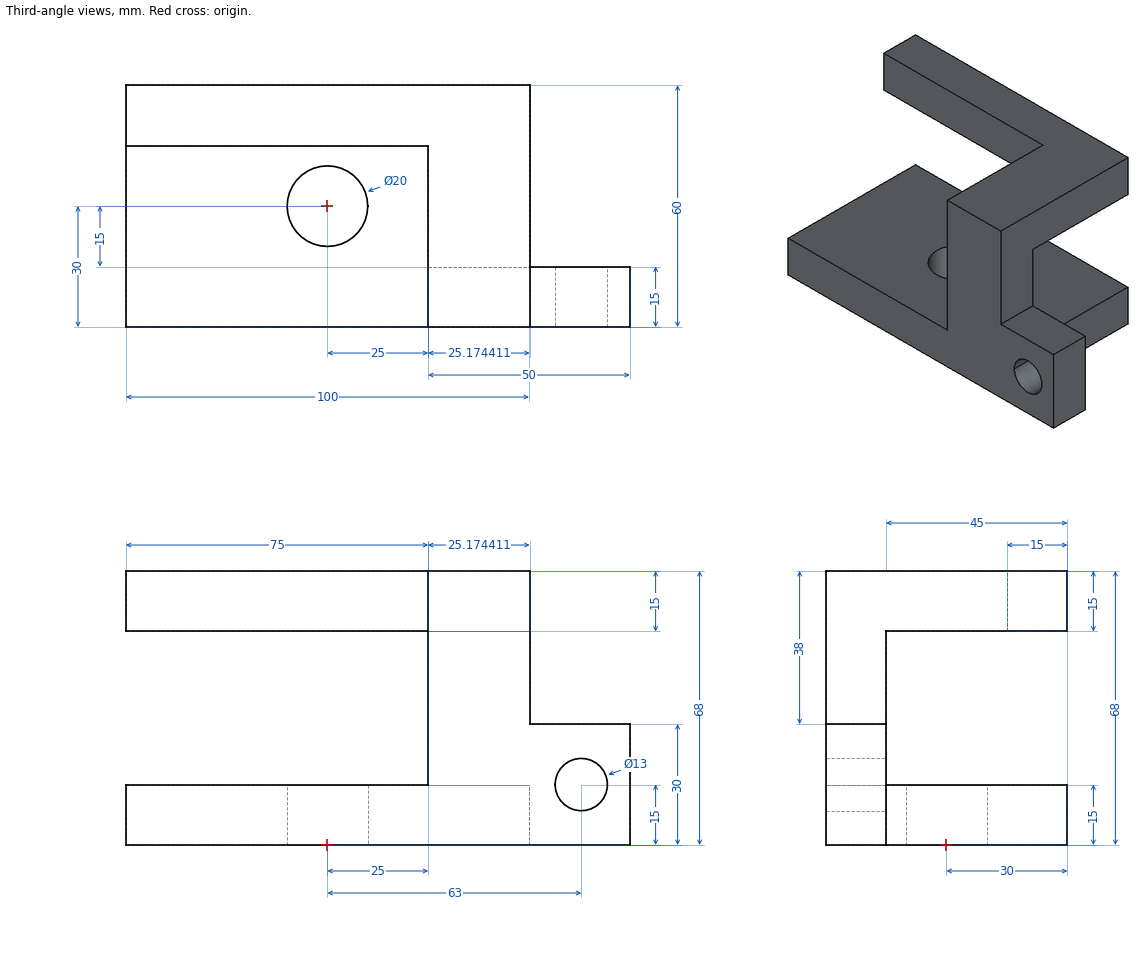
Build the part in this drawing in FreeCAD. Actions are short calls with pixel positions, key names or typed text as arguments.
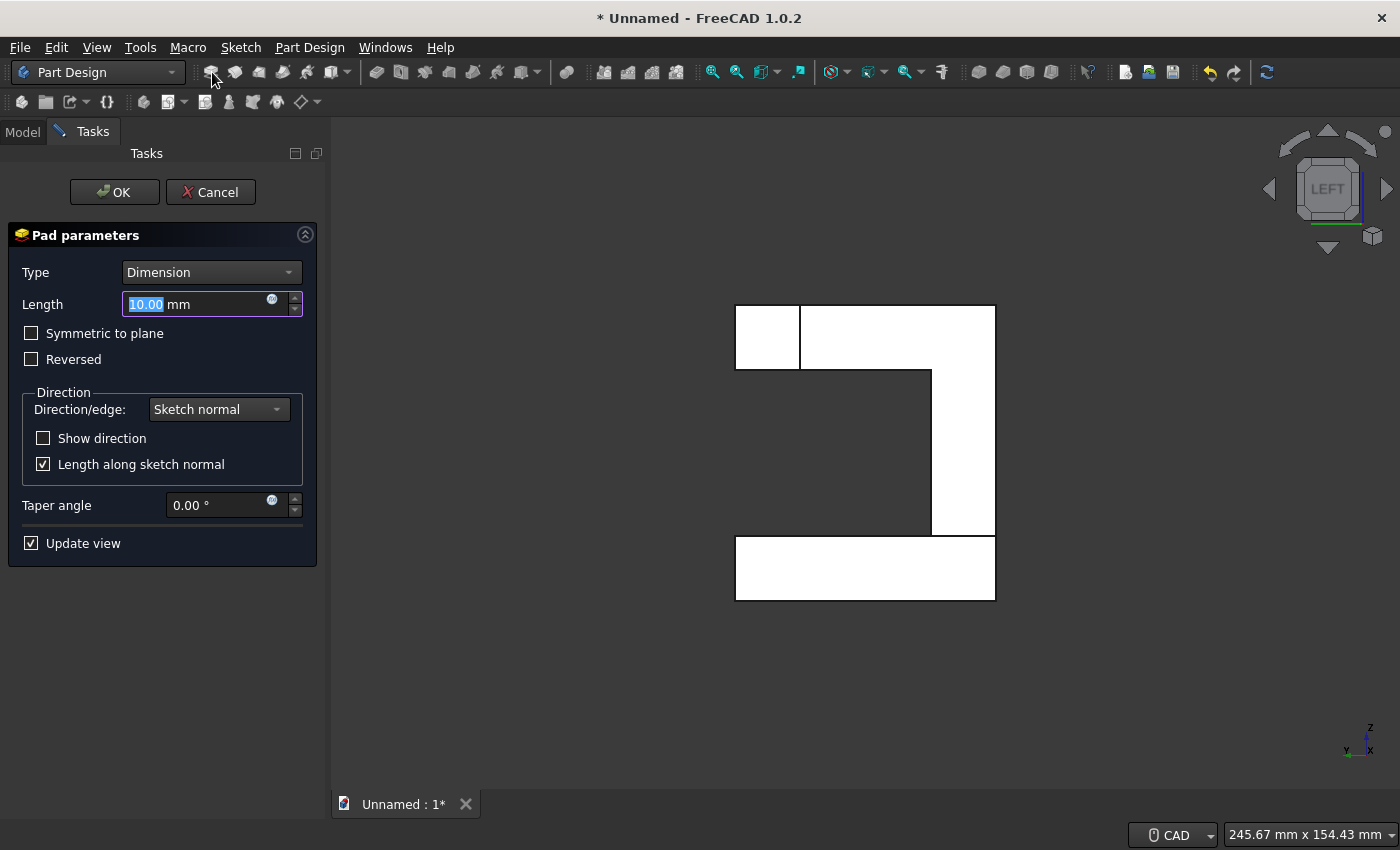
text(75)
key(Tab)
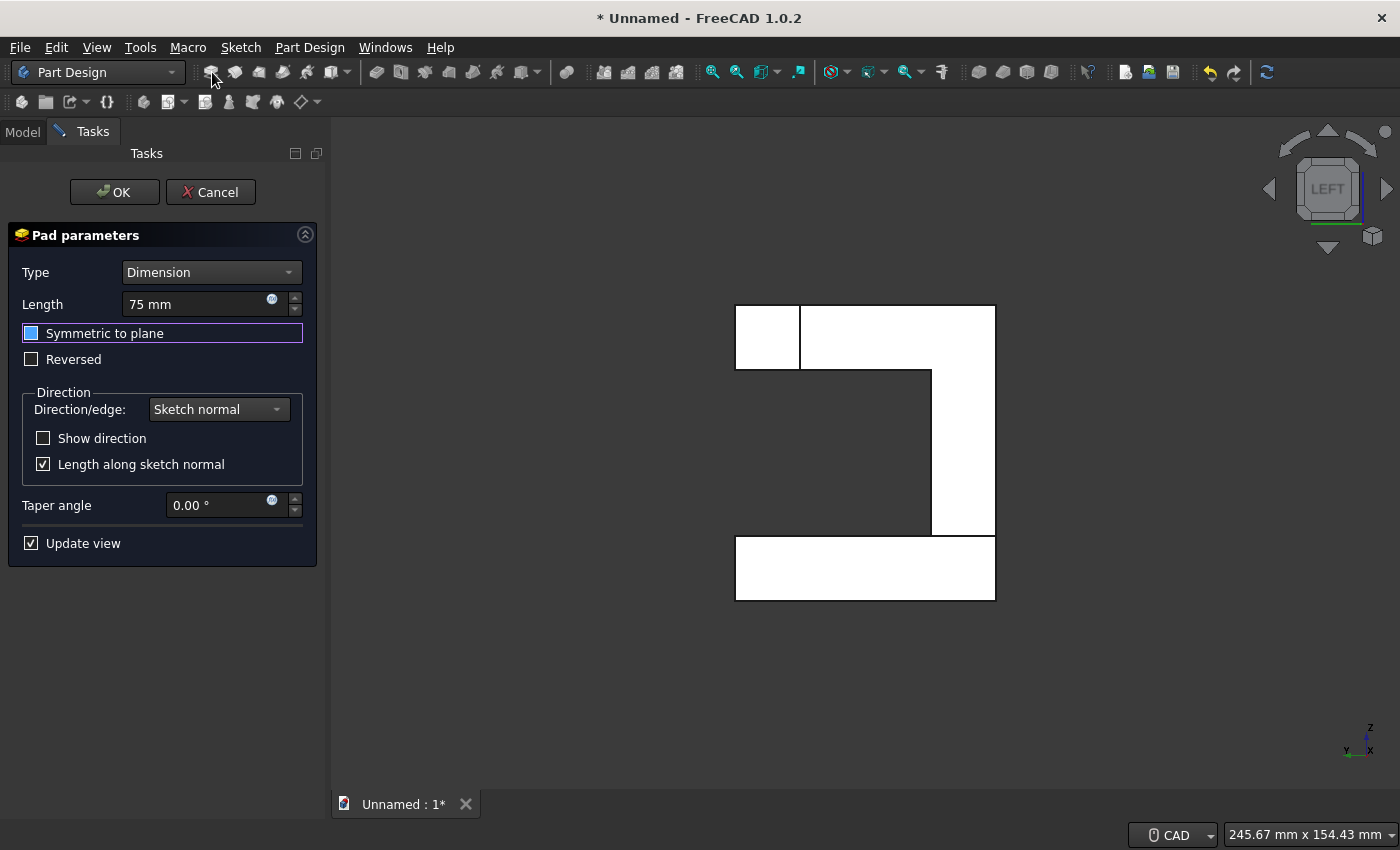
click(115, 192)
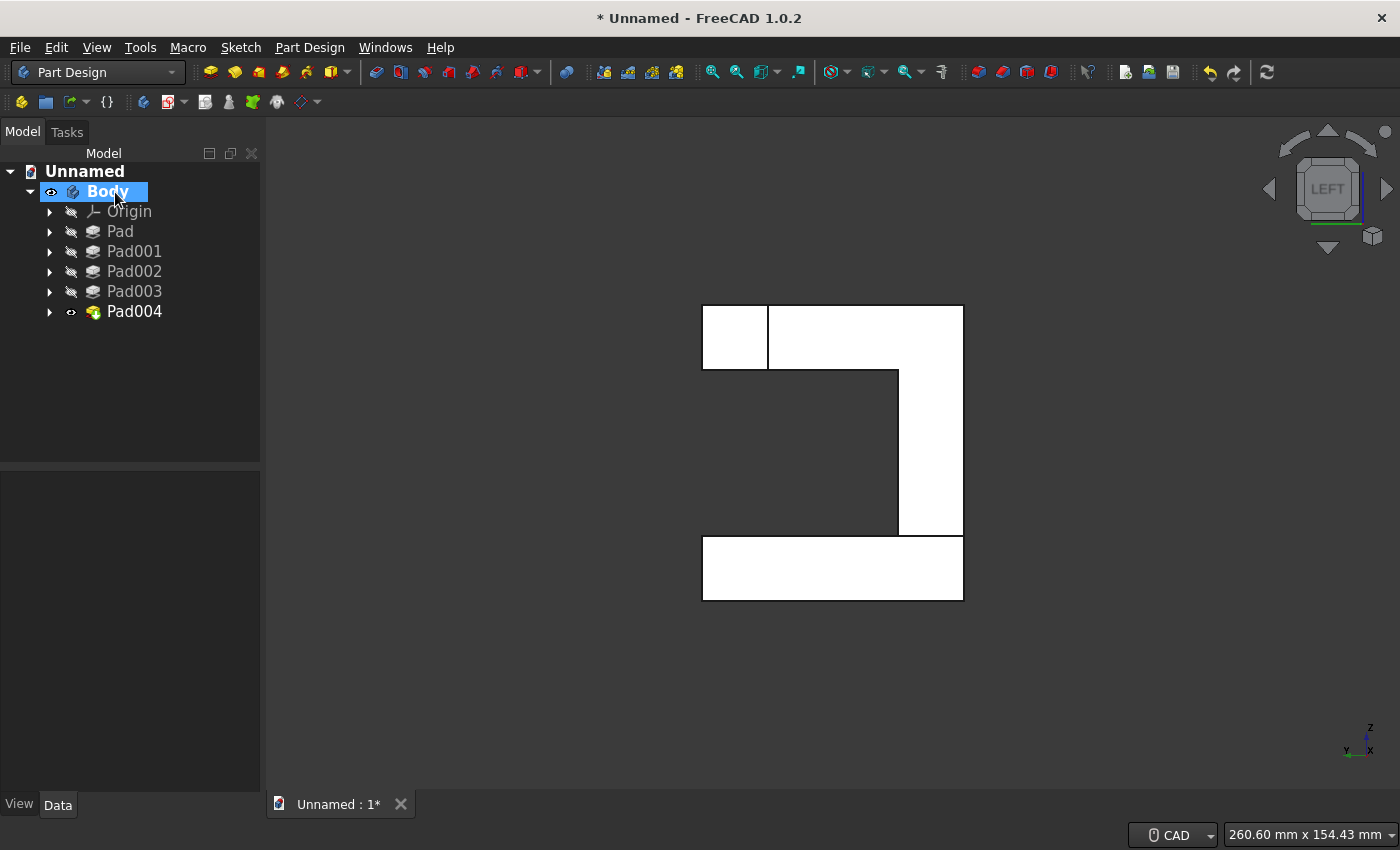
click(714, 72)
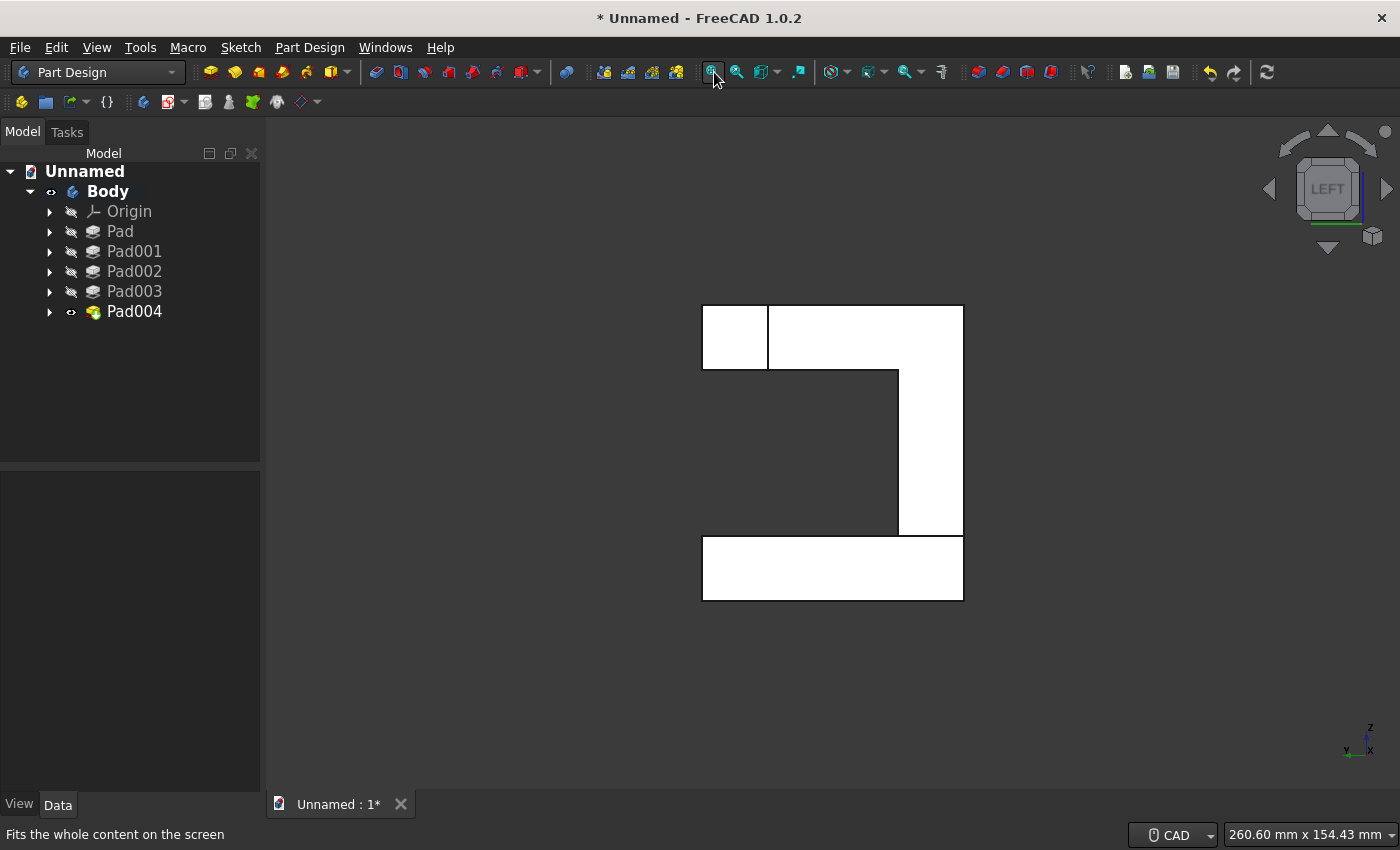
key(4)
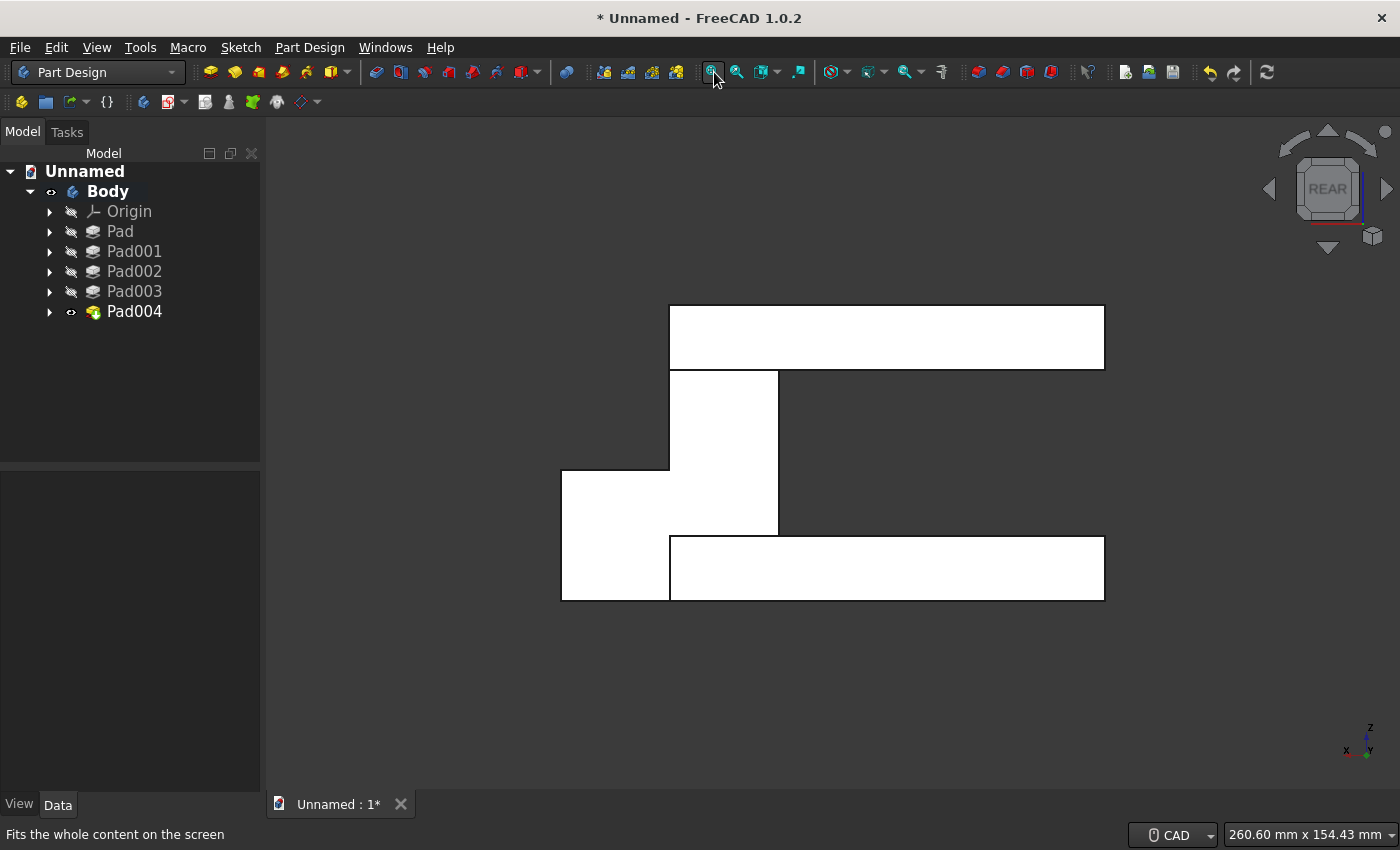
click(608, 518)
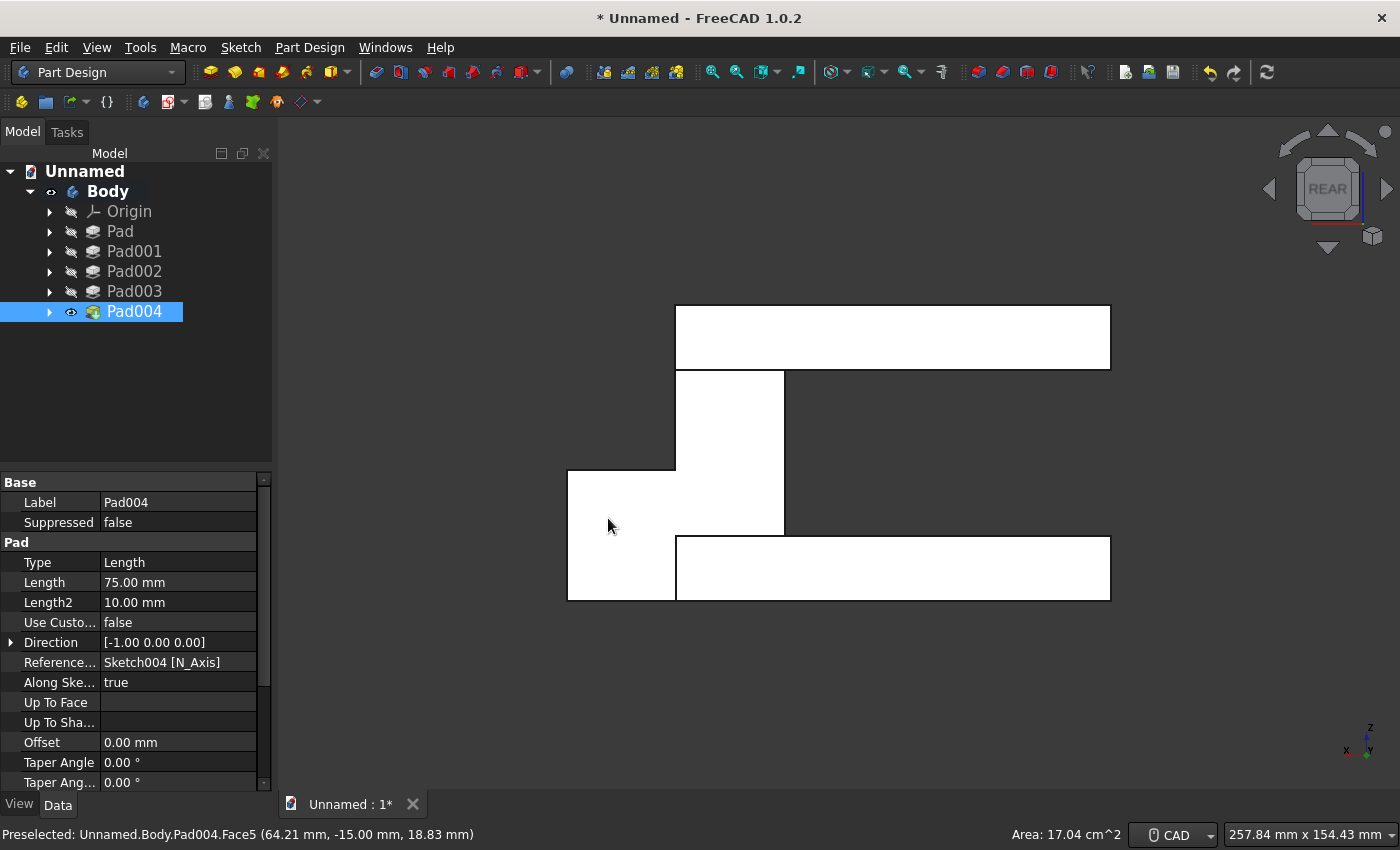
click(168, 102)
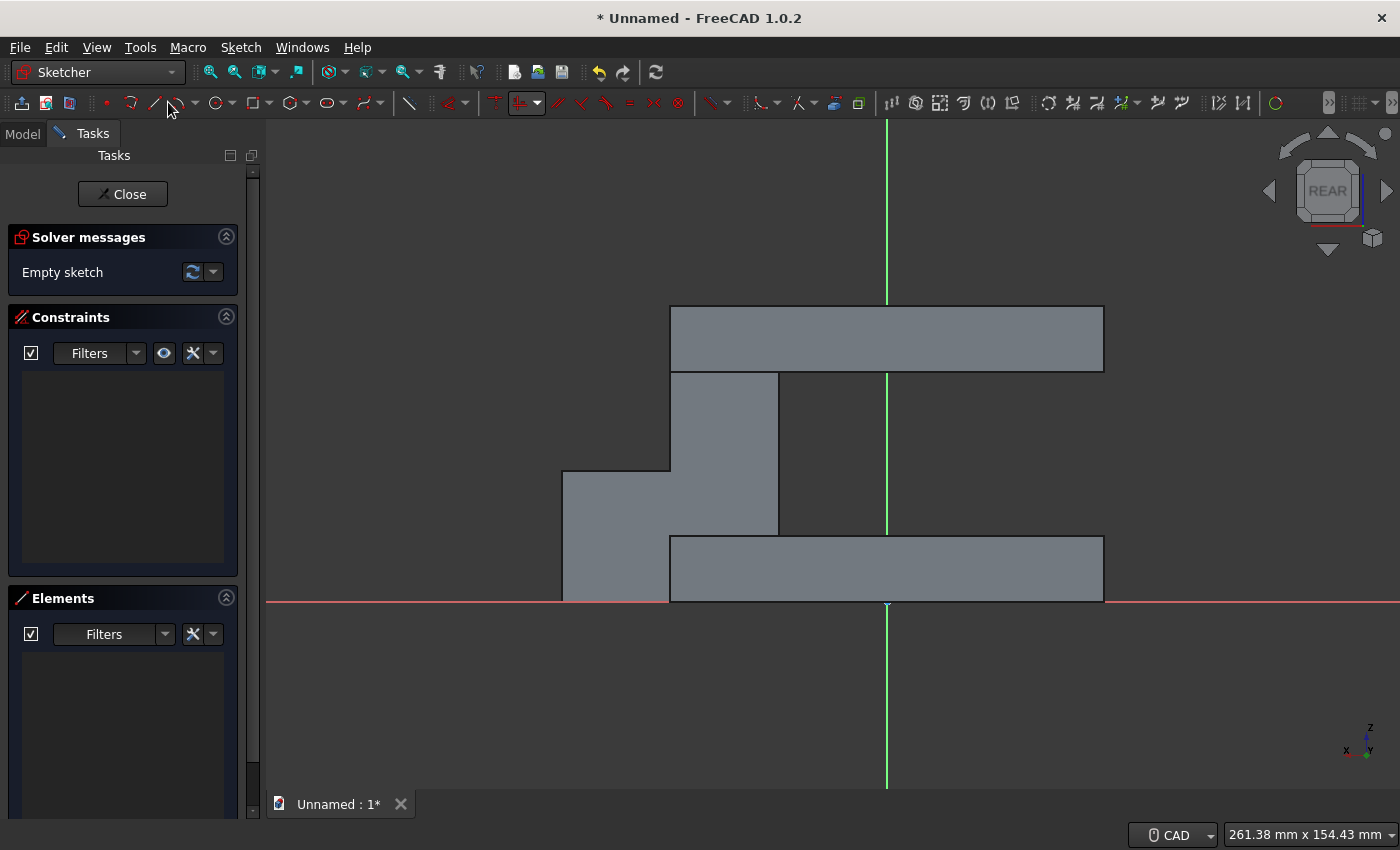
scroll(590, 549, up, 10)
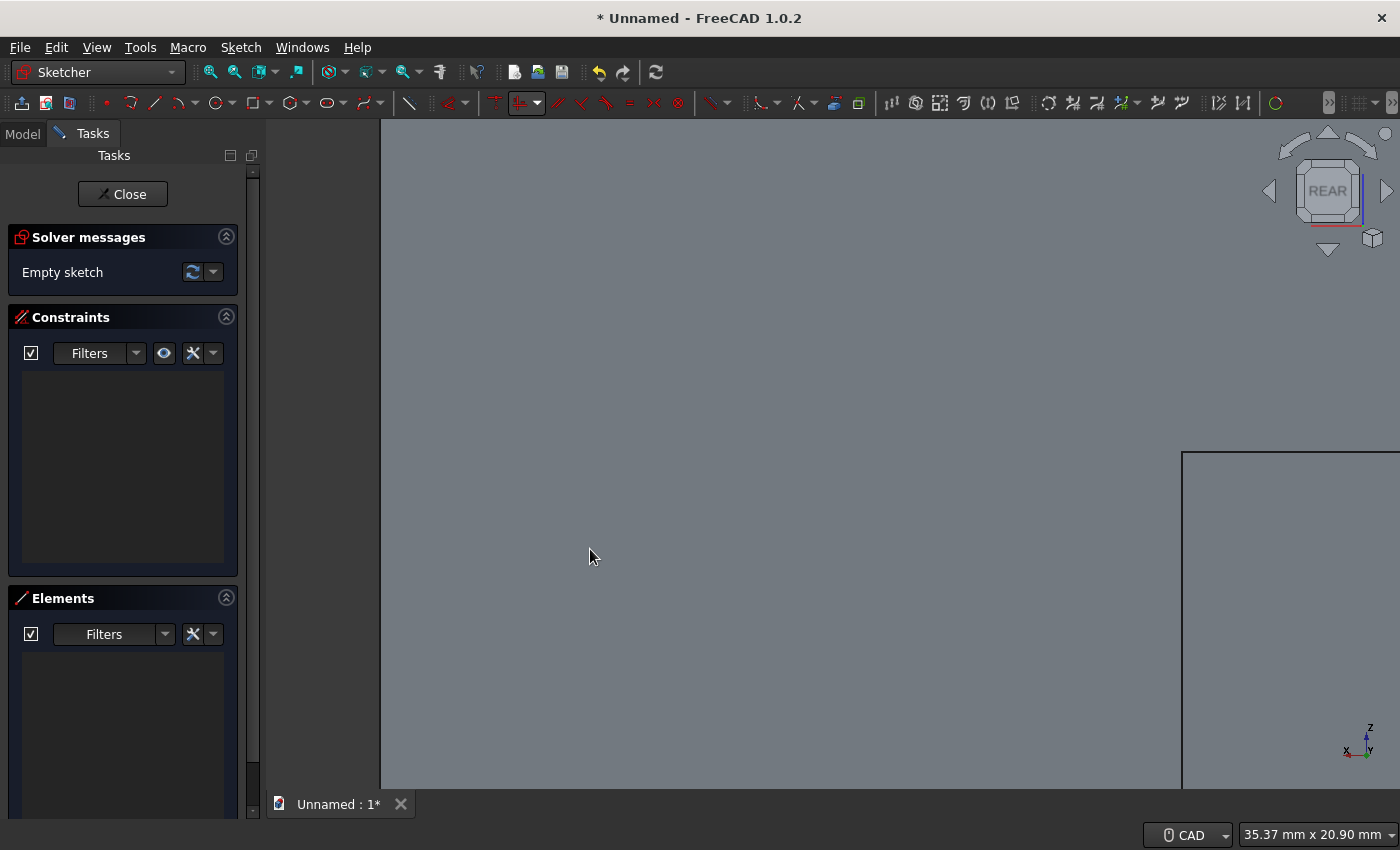
click(216, 104)